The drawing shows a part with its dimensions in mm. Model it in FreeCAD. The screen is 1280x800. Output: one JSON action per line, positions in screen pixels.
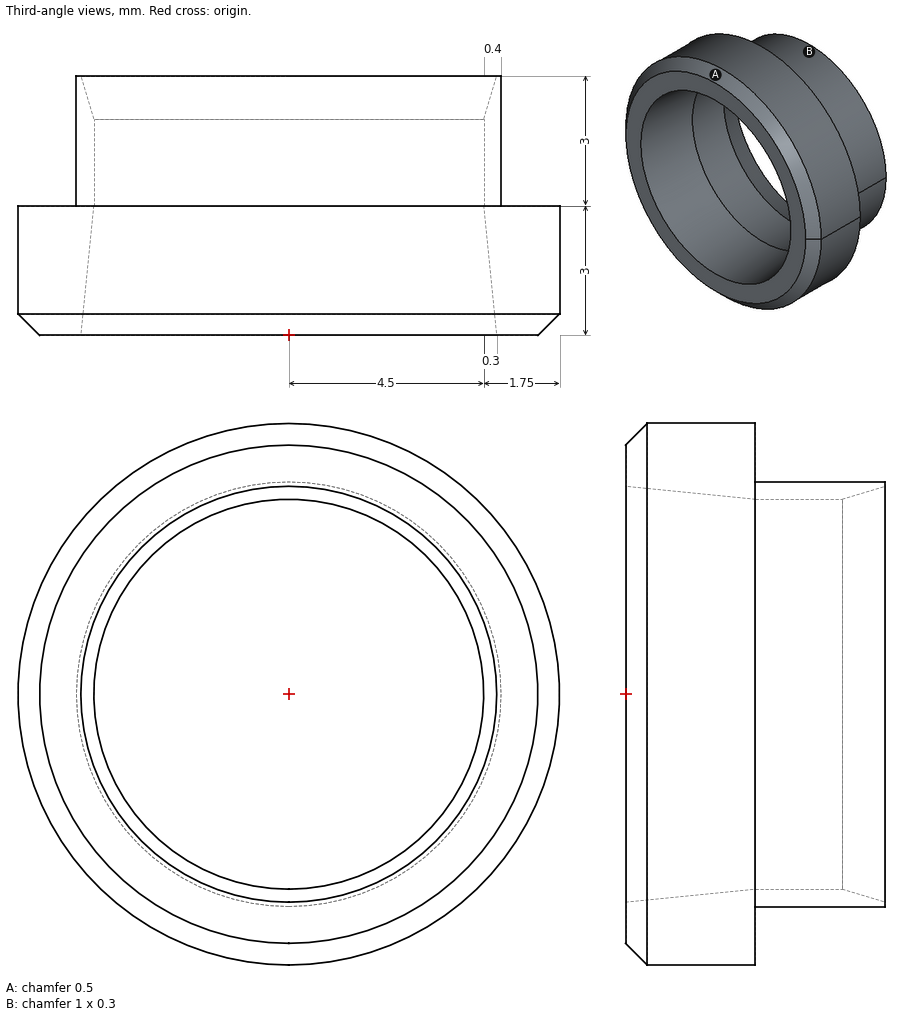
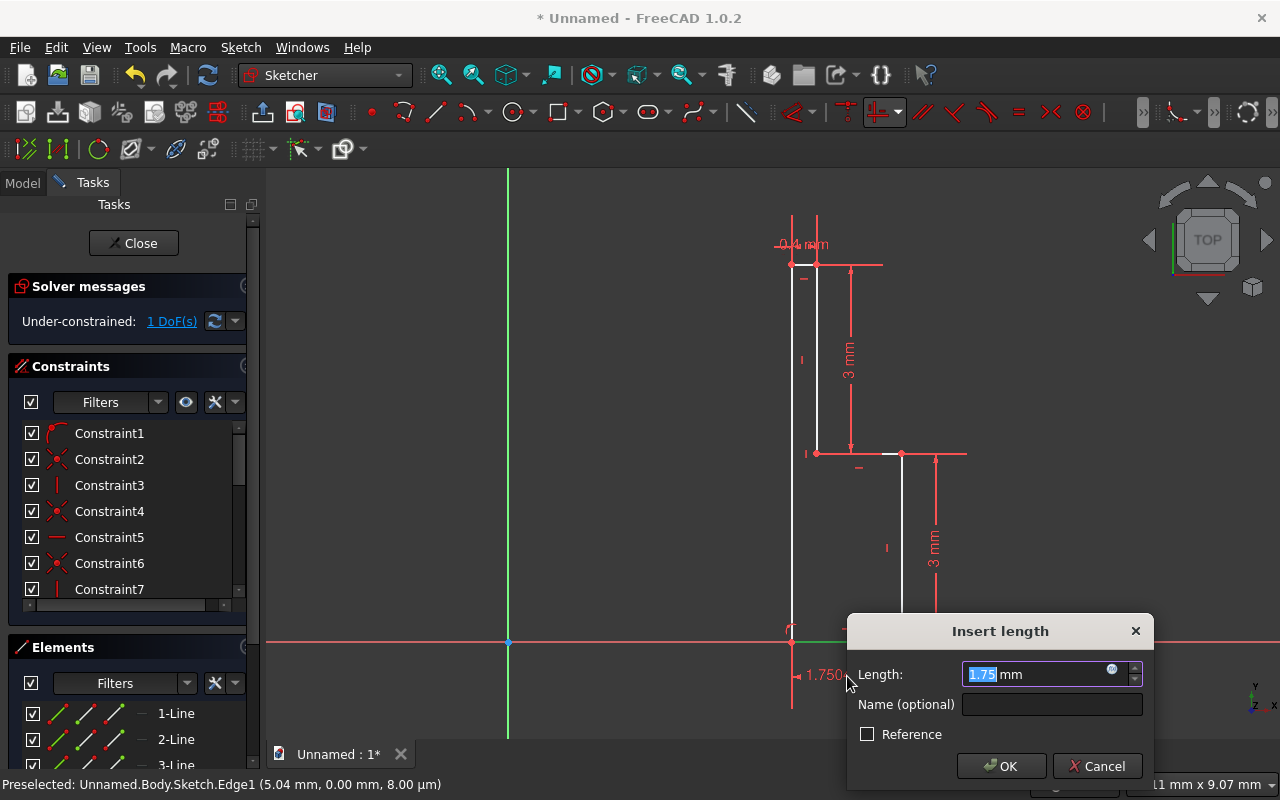
{"action": "type", "text": "1.75"}
{"action": "key", "text": "Return"}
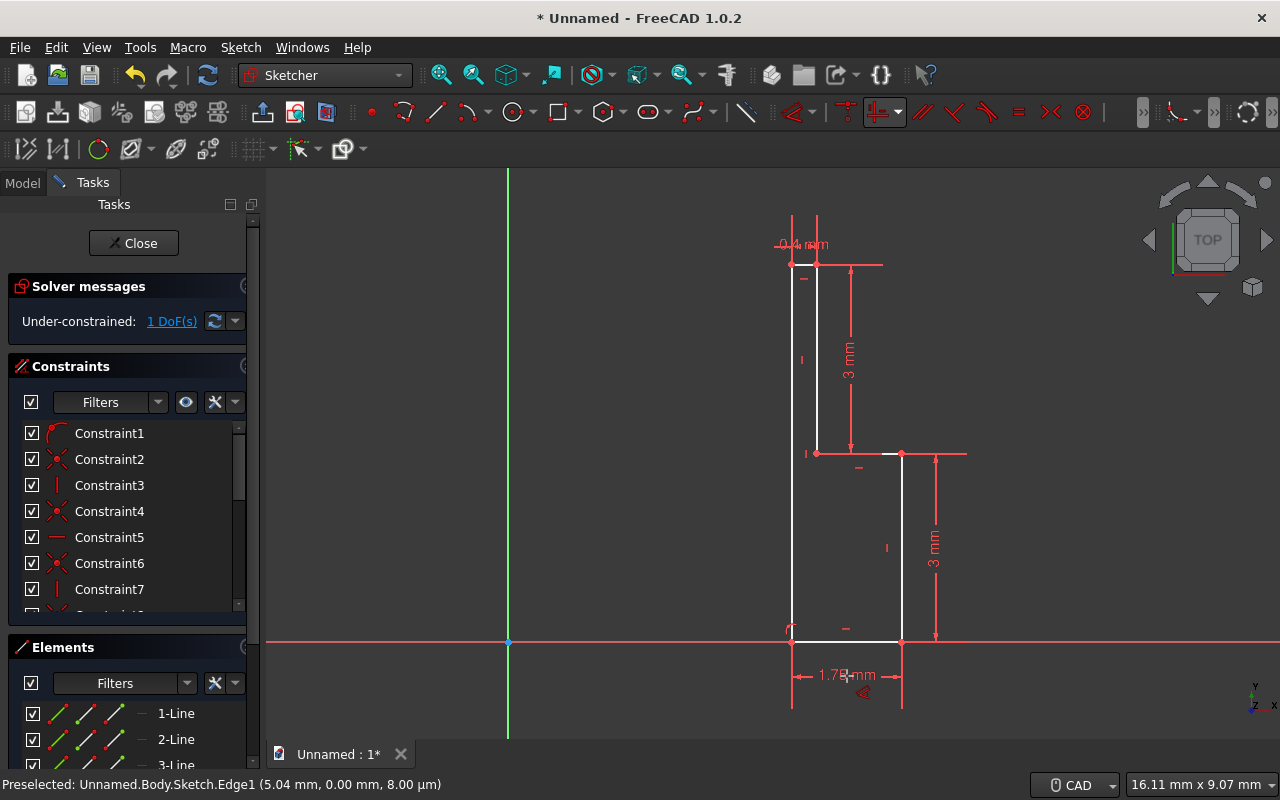
{"action": "left_click", "coordinate": [792, 642]}
{"action": "left_click", "coordinate": [650, 676]}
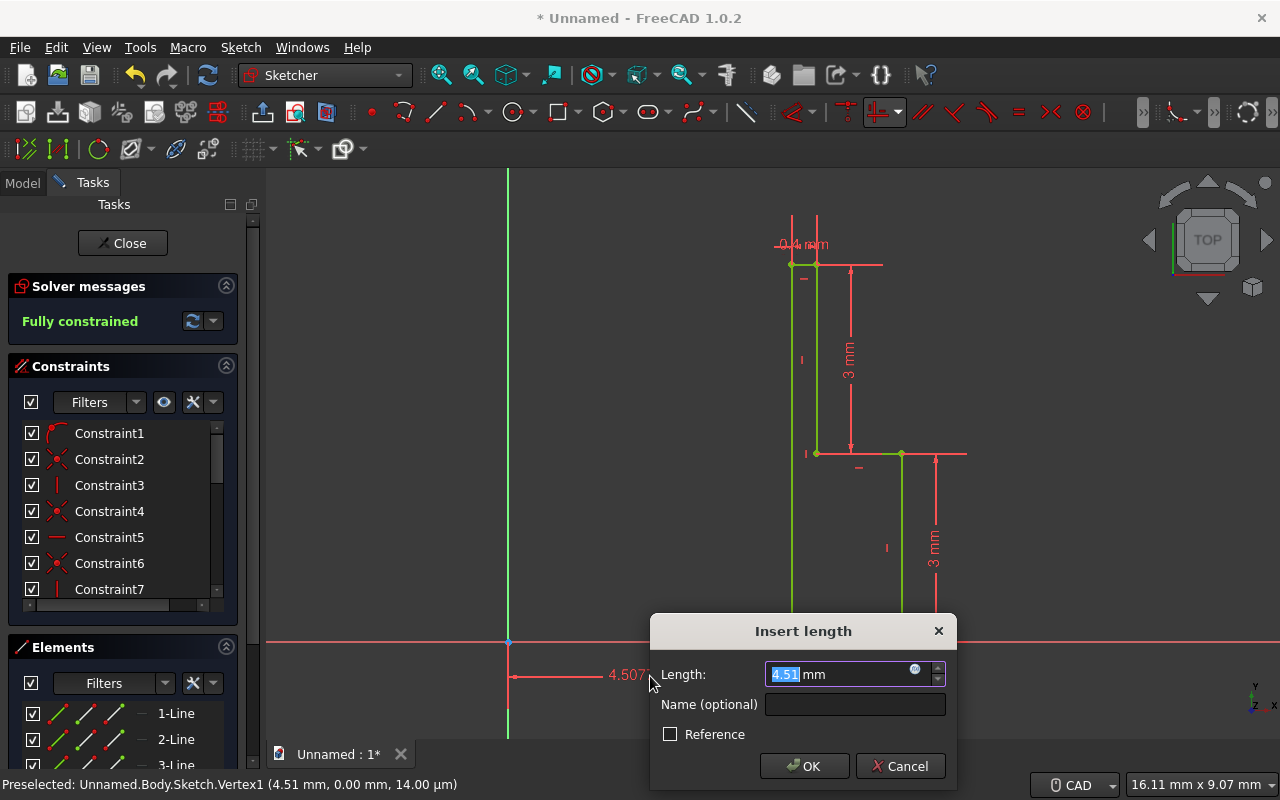
{"action": "type", "text": "4.5"}
{"action": "key", "text": "Return"}
{"action": "key", "text": "Escape"}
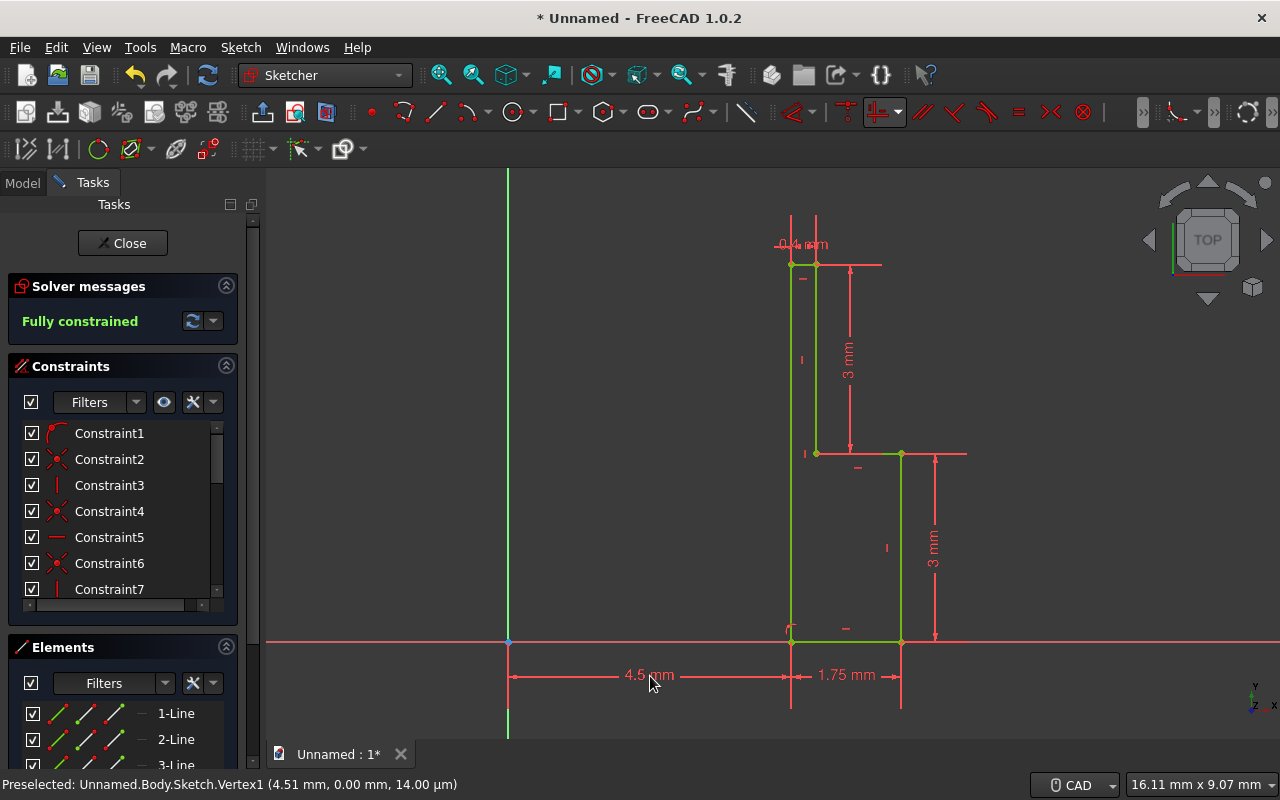
{"action": "left_click", "coordinate": [123, 243]}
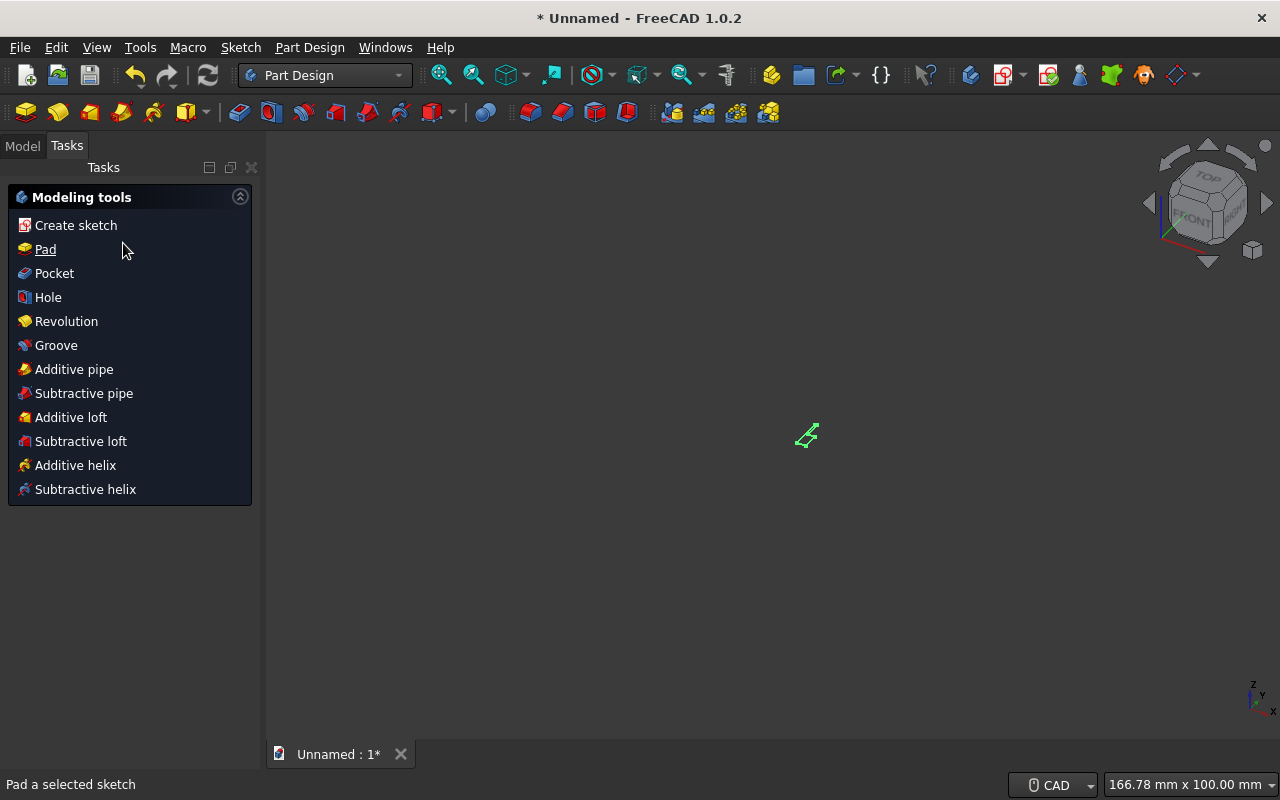
{"action": "left_click", "coordinate": [58, 112]}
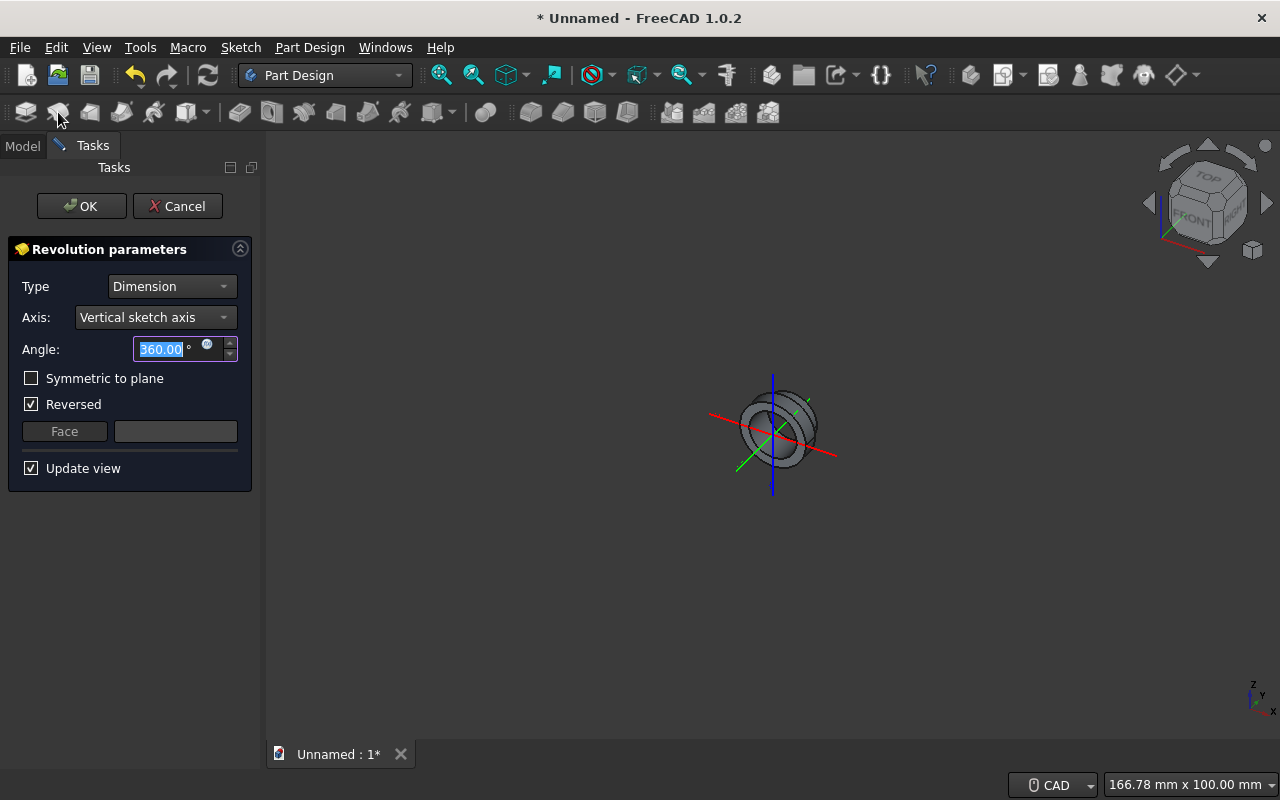
{"action": "left_click", "coordinate": [82, 206]}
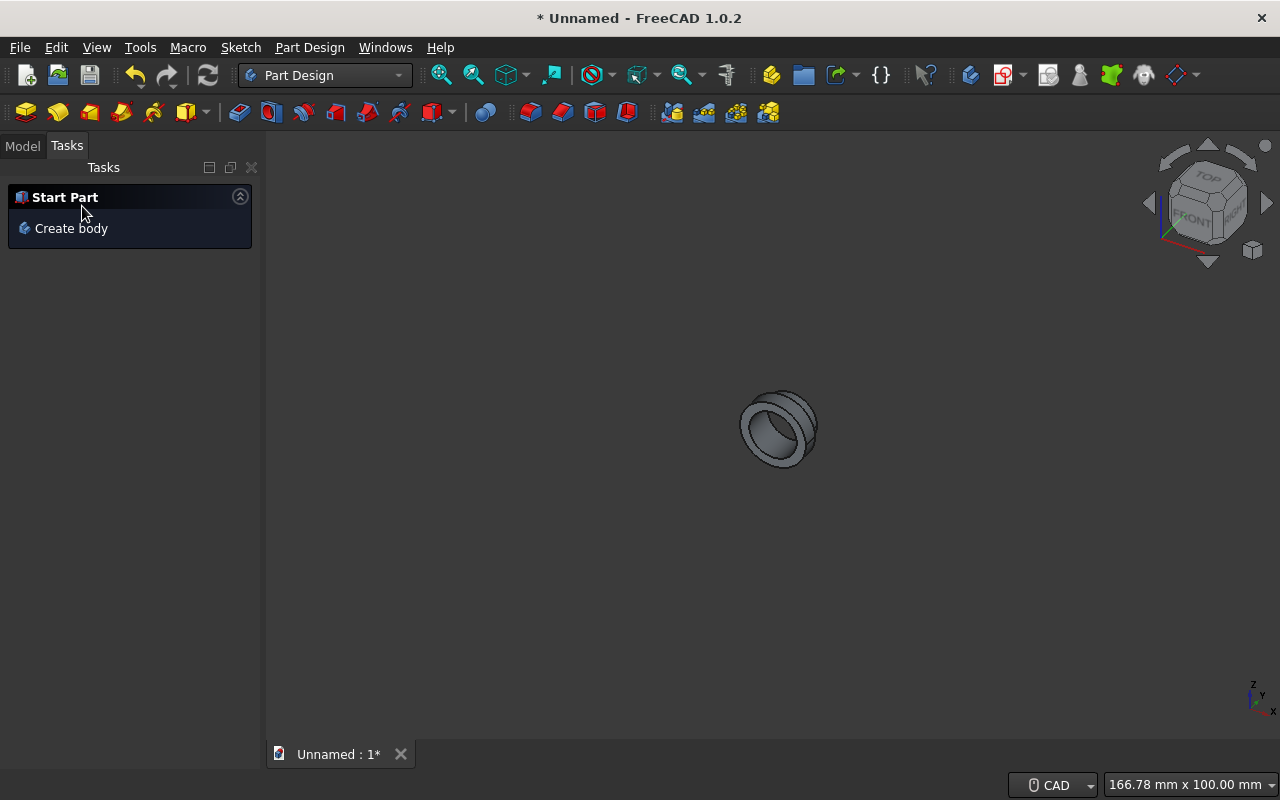
{"action": "key", "text": "v f"}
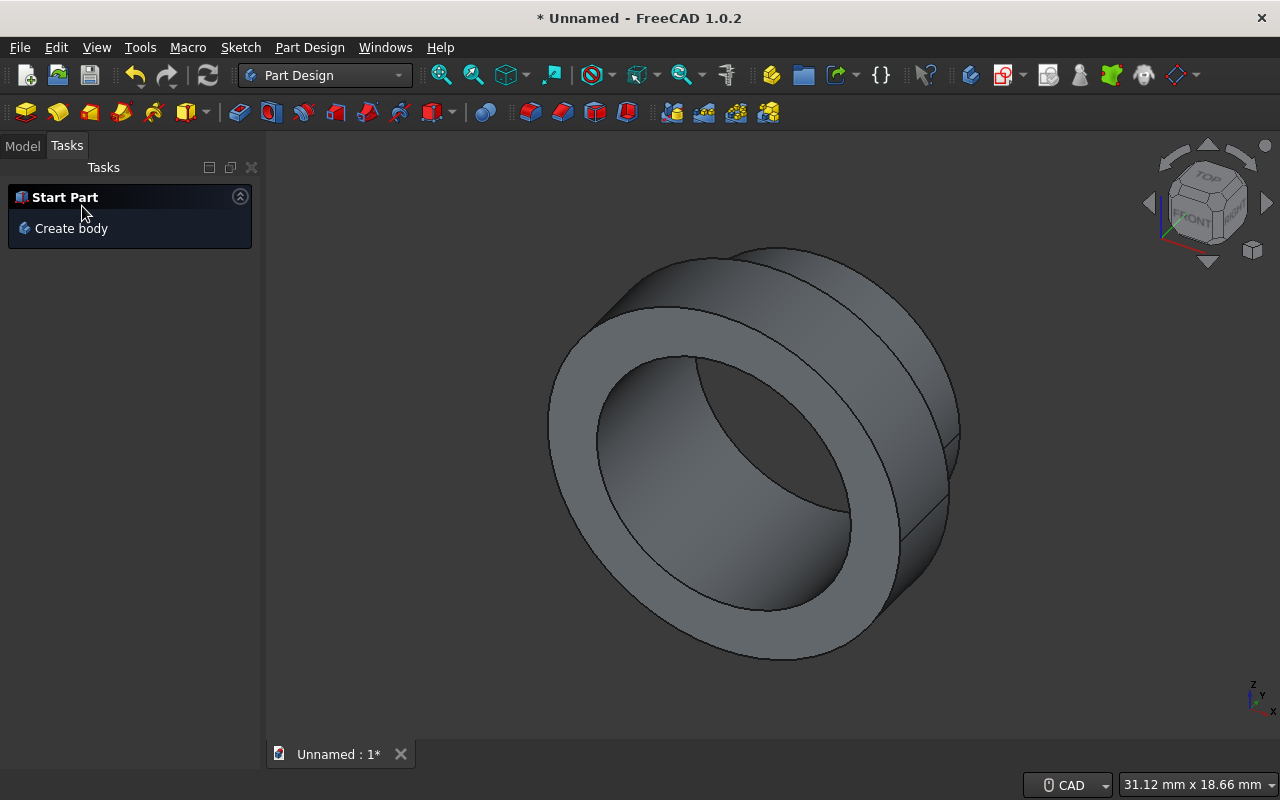
{"action": "left_click", "coordinate": [1004, 76]}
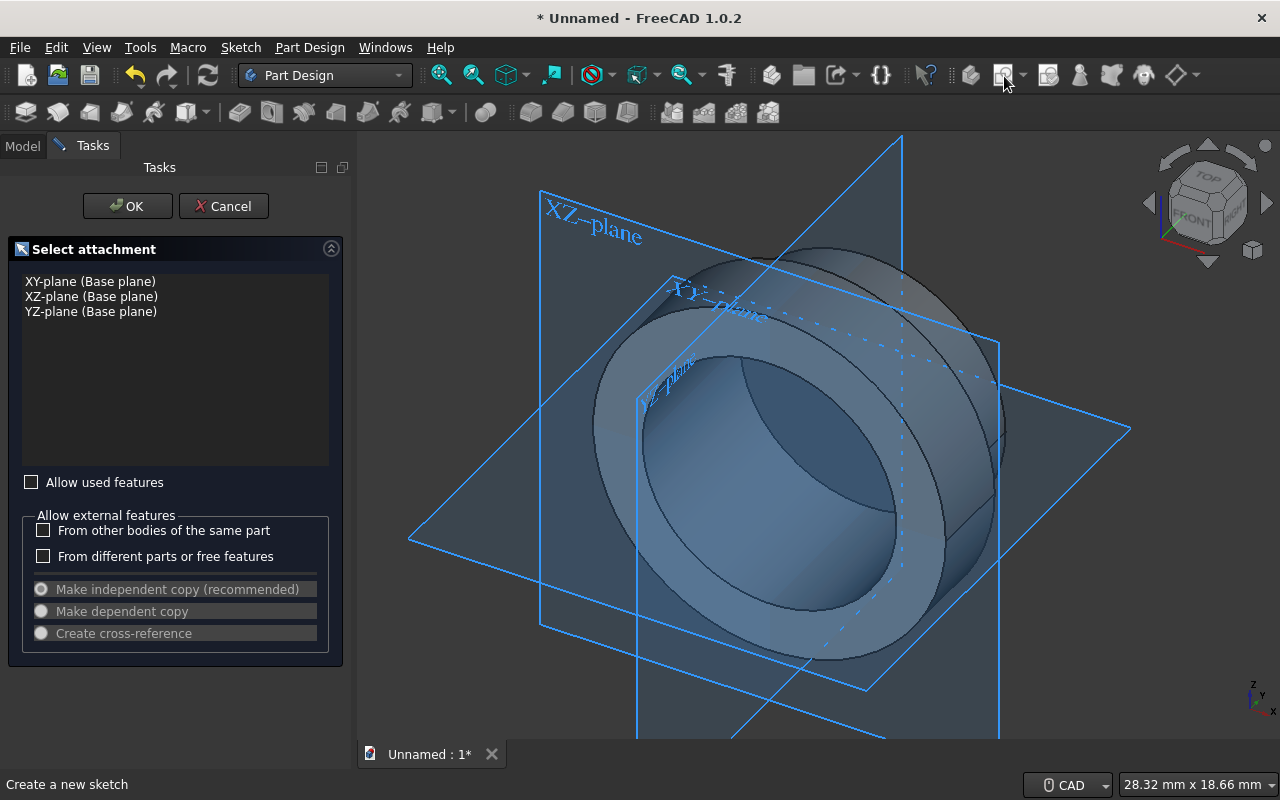
{"action": "left_click", "coordinate": [82, 282]}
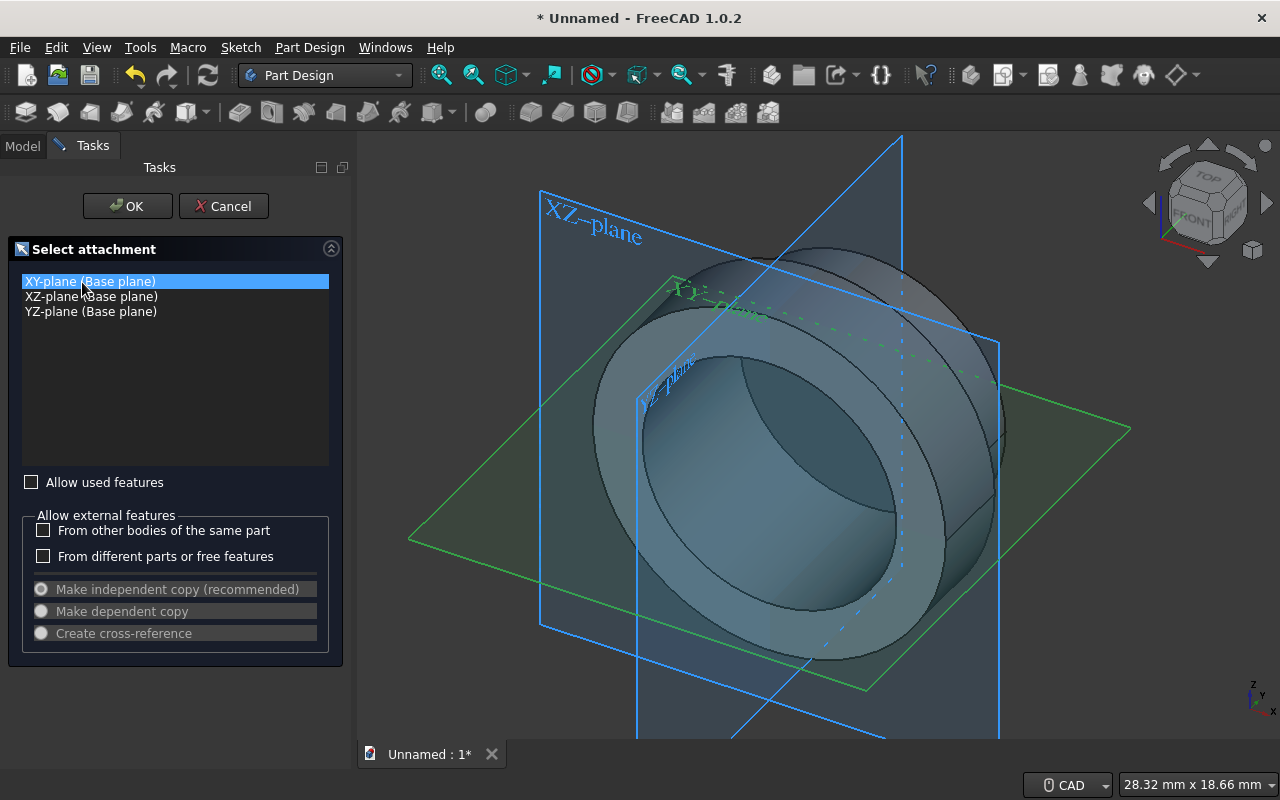
{"action": "left_click", "coordinate": [128, 206]}